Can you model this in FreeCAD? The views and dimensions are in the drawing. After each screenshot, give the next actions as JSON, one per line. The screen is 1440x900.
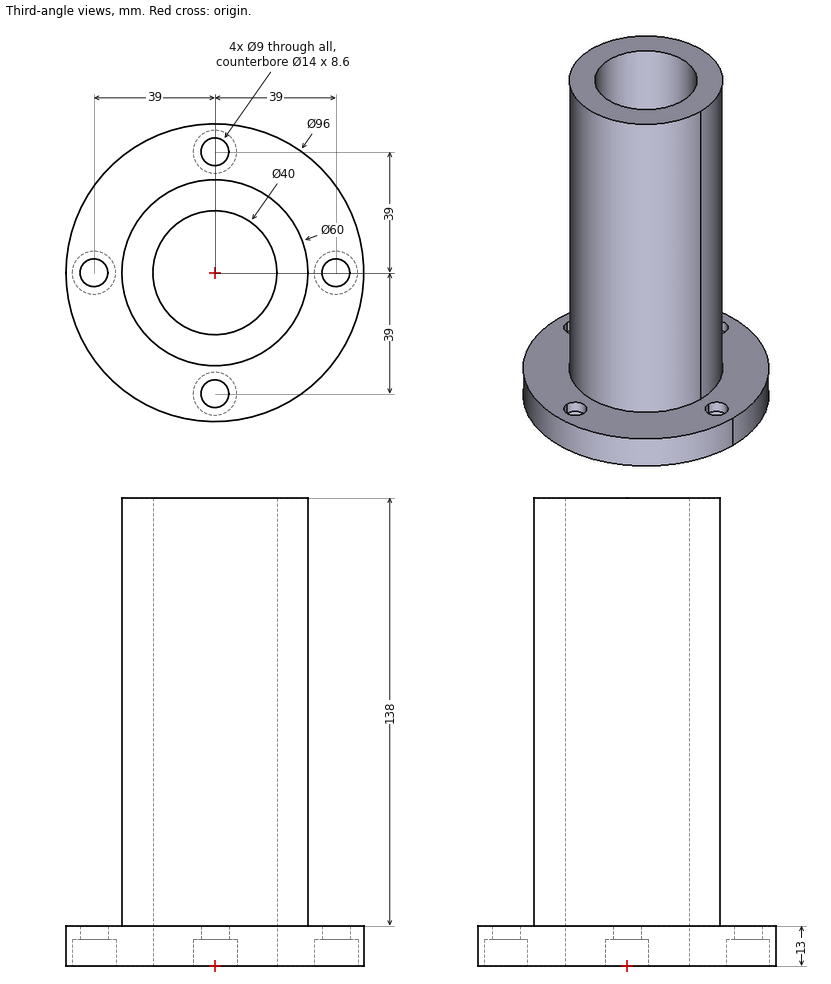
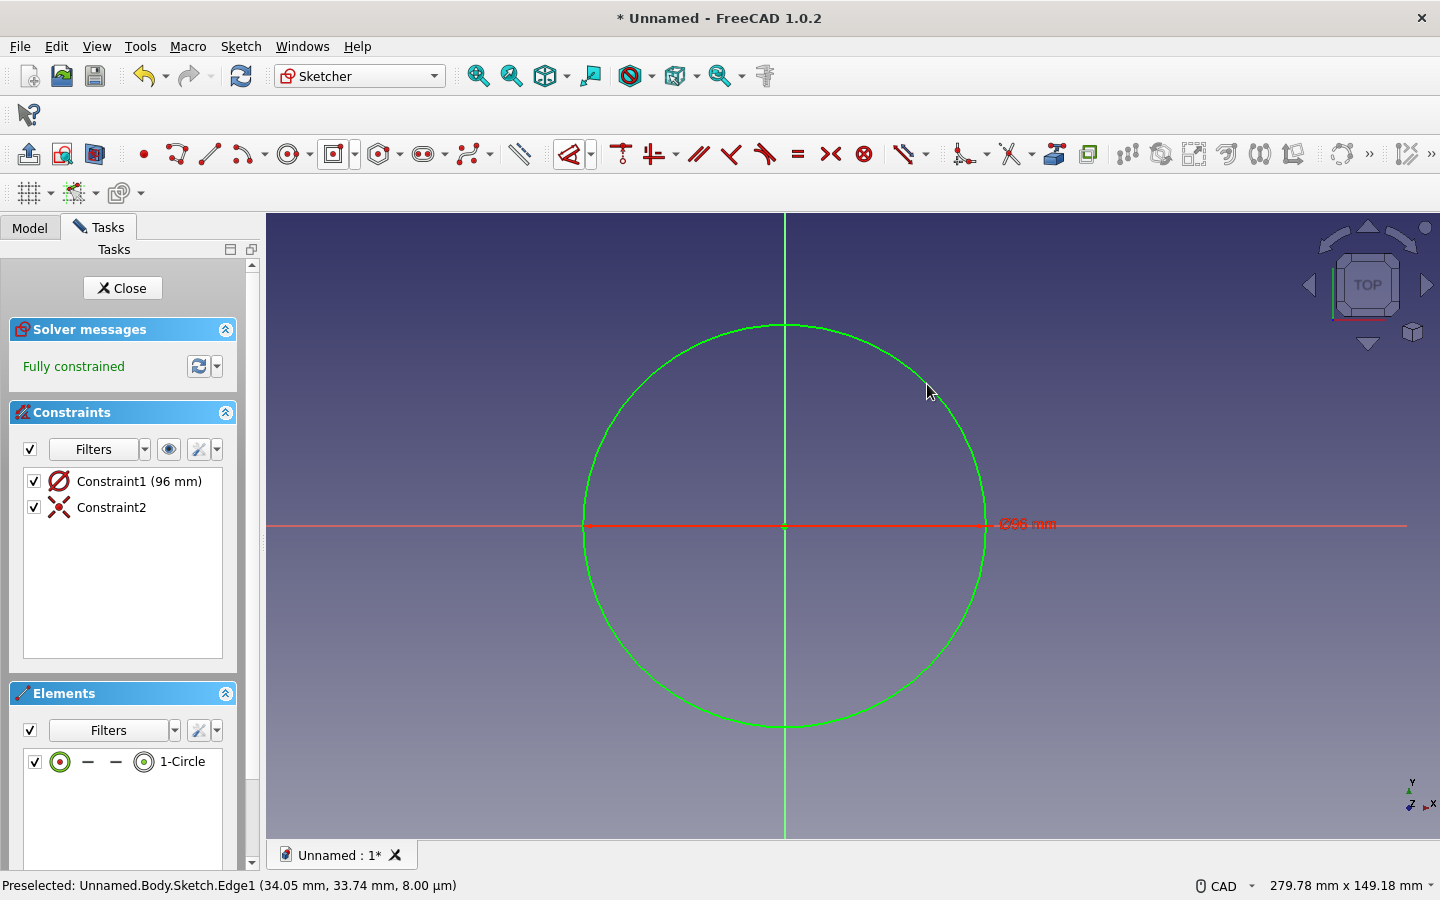
{"action": "left_click", "coordinate": [123, 288]}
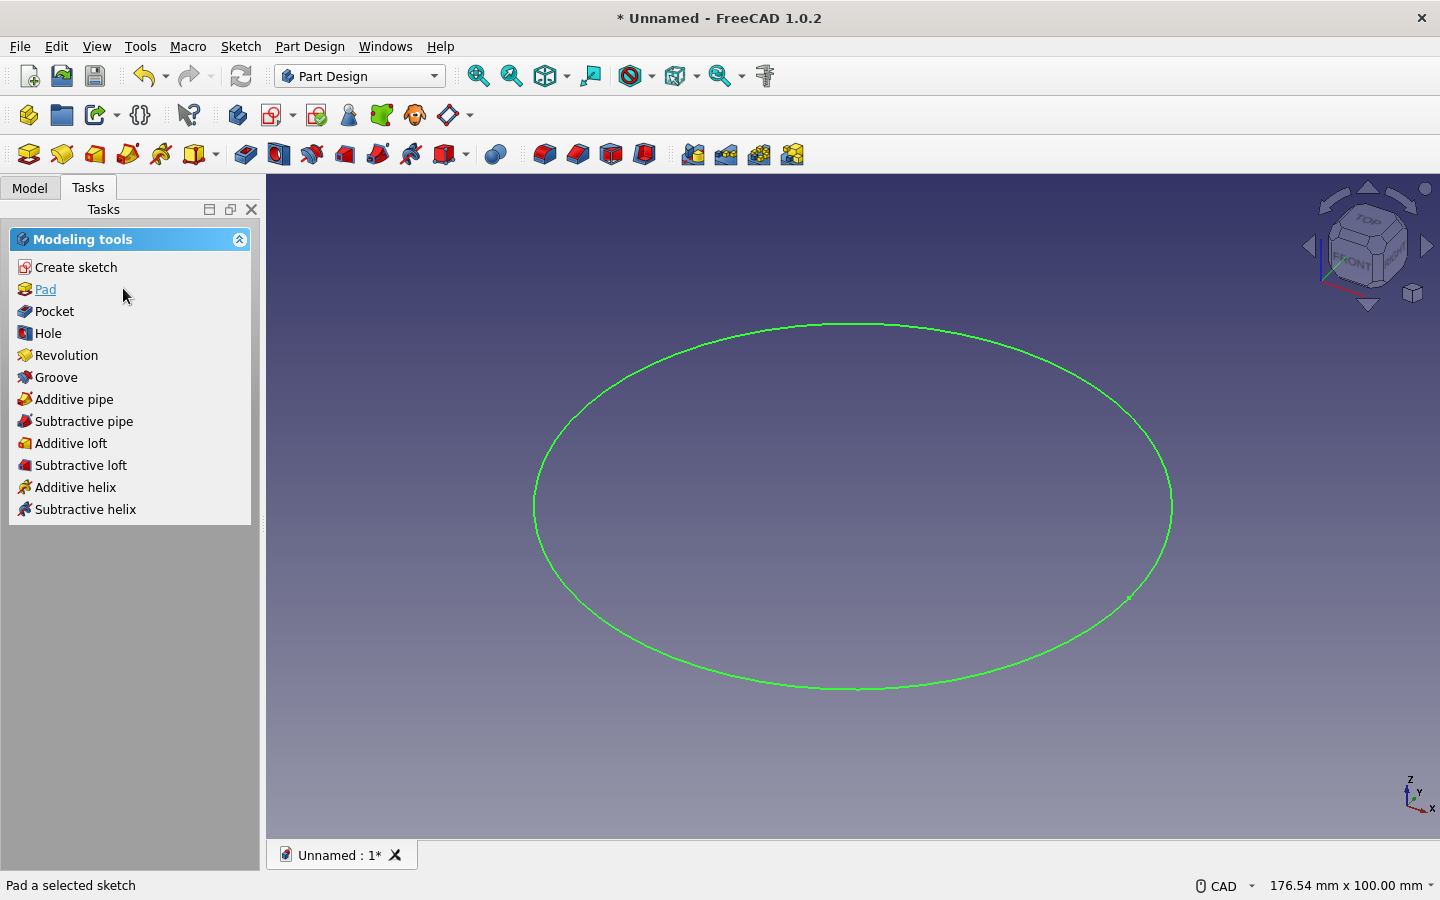
{"action": "left_click", "coordinate": [29, 154]}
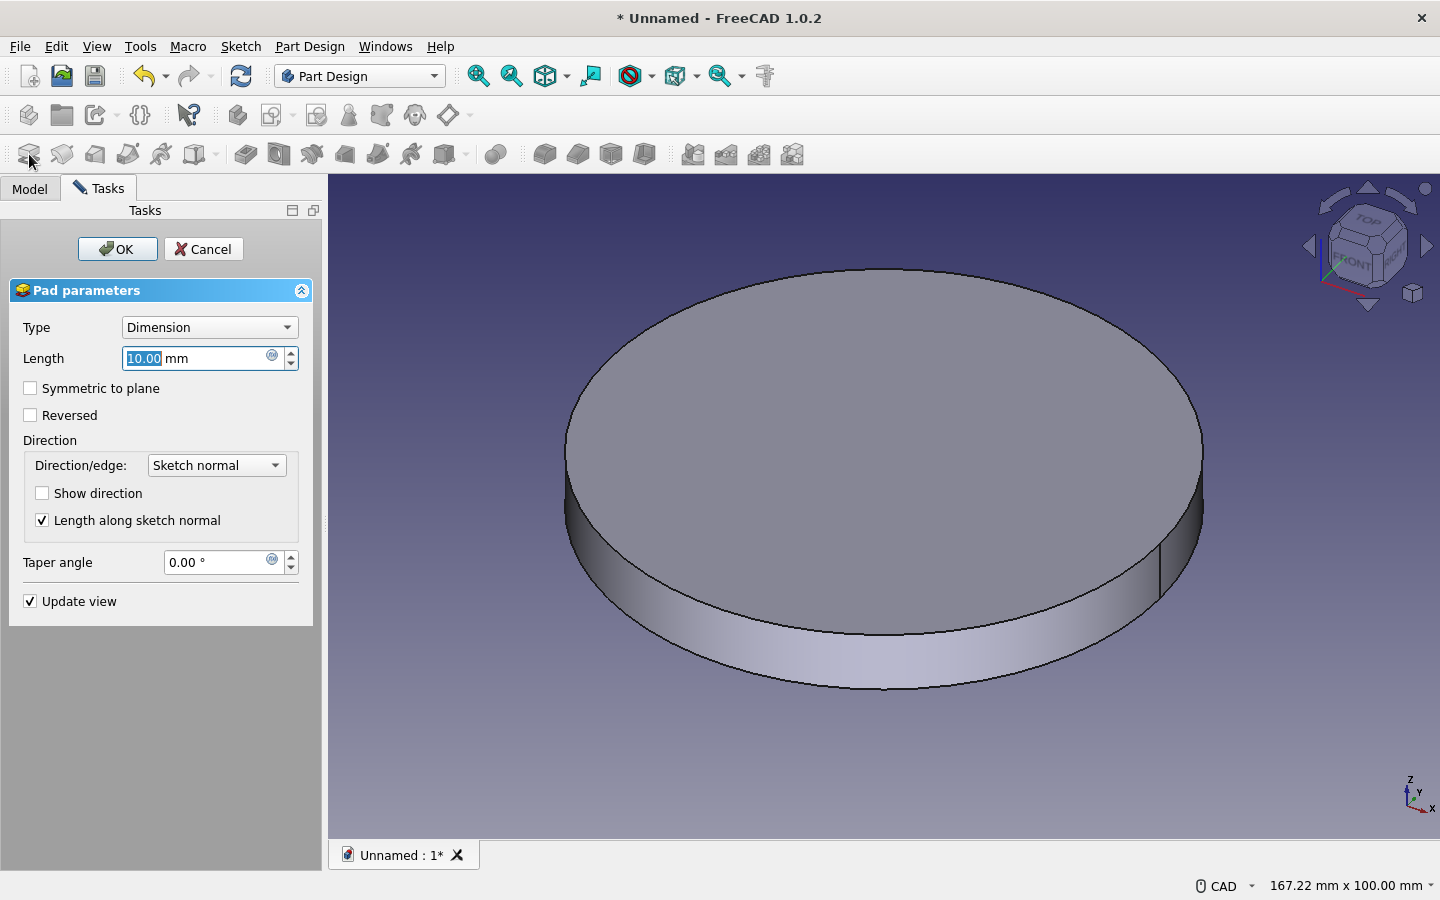
{"action": "type", "text": "13"}
{"action": "key", "text": "Tab"}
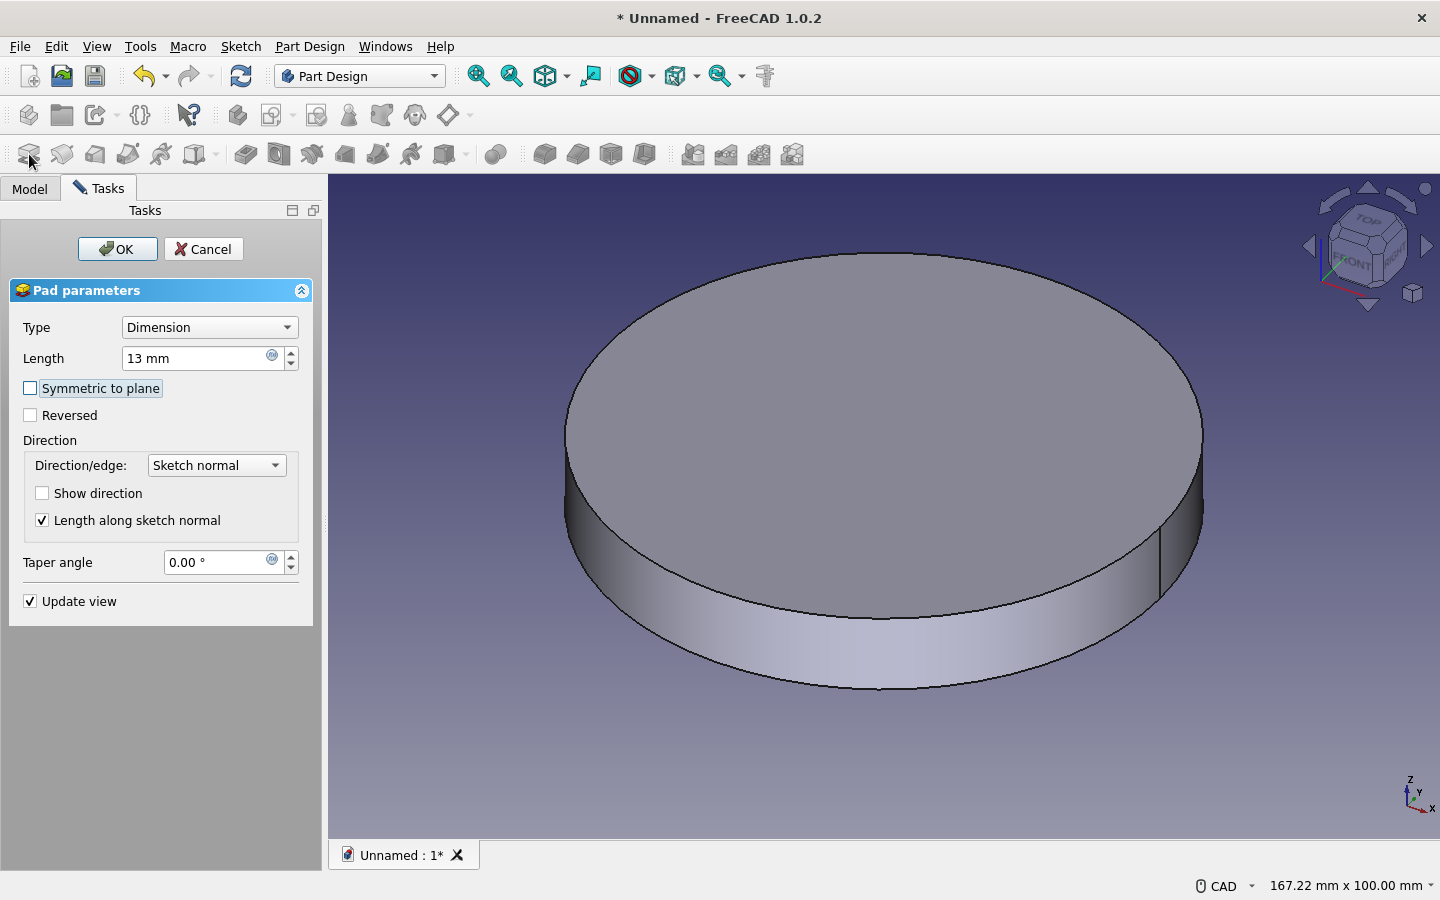
{"action": "left_click", "coordinate": [118, 249]}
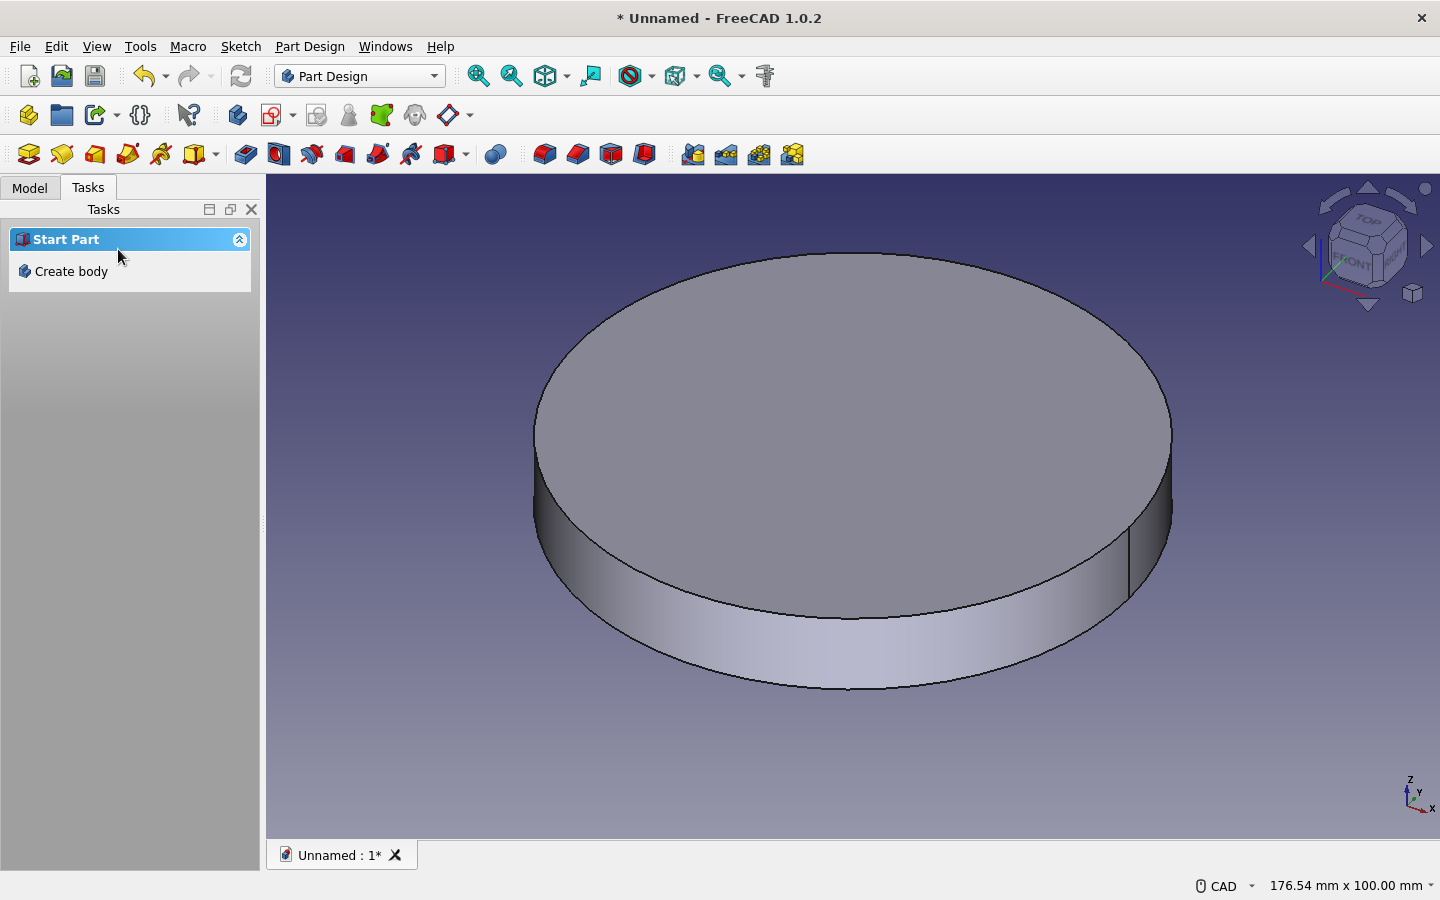
{"action": "left_click", "coordinate": [270, 116]}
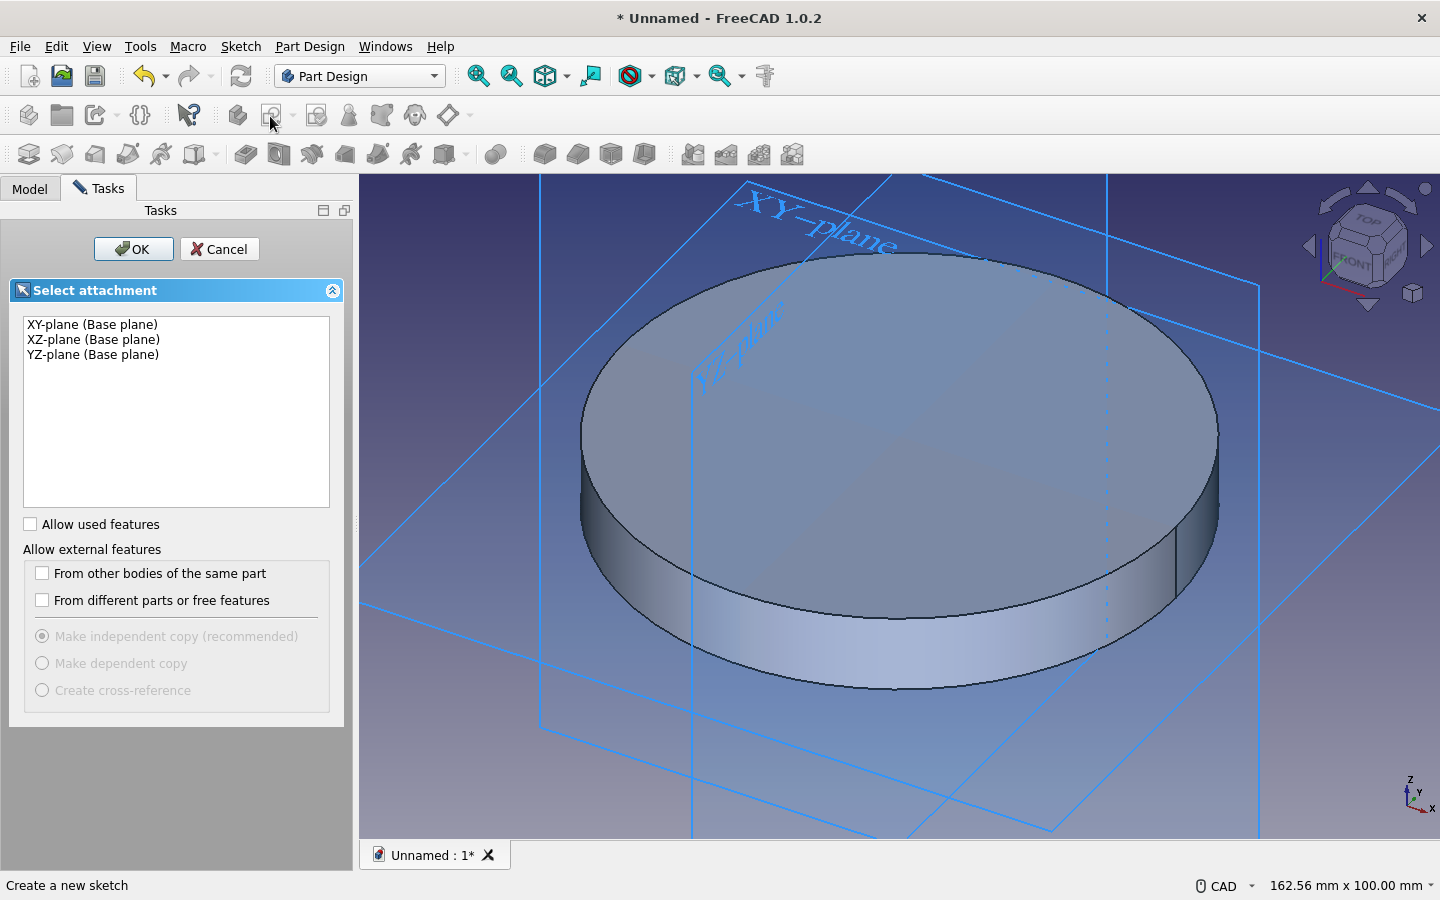
{"action": "left_click", "coordinate": [84, 324]}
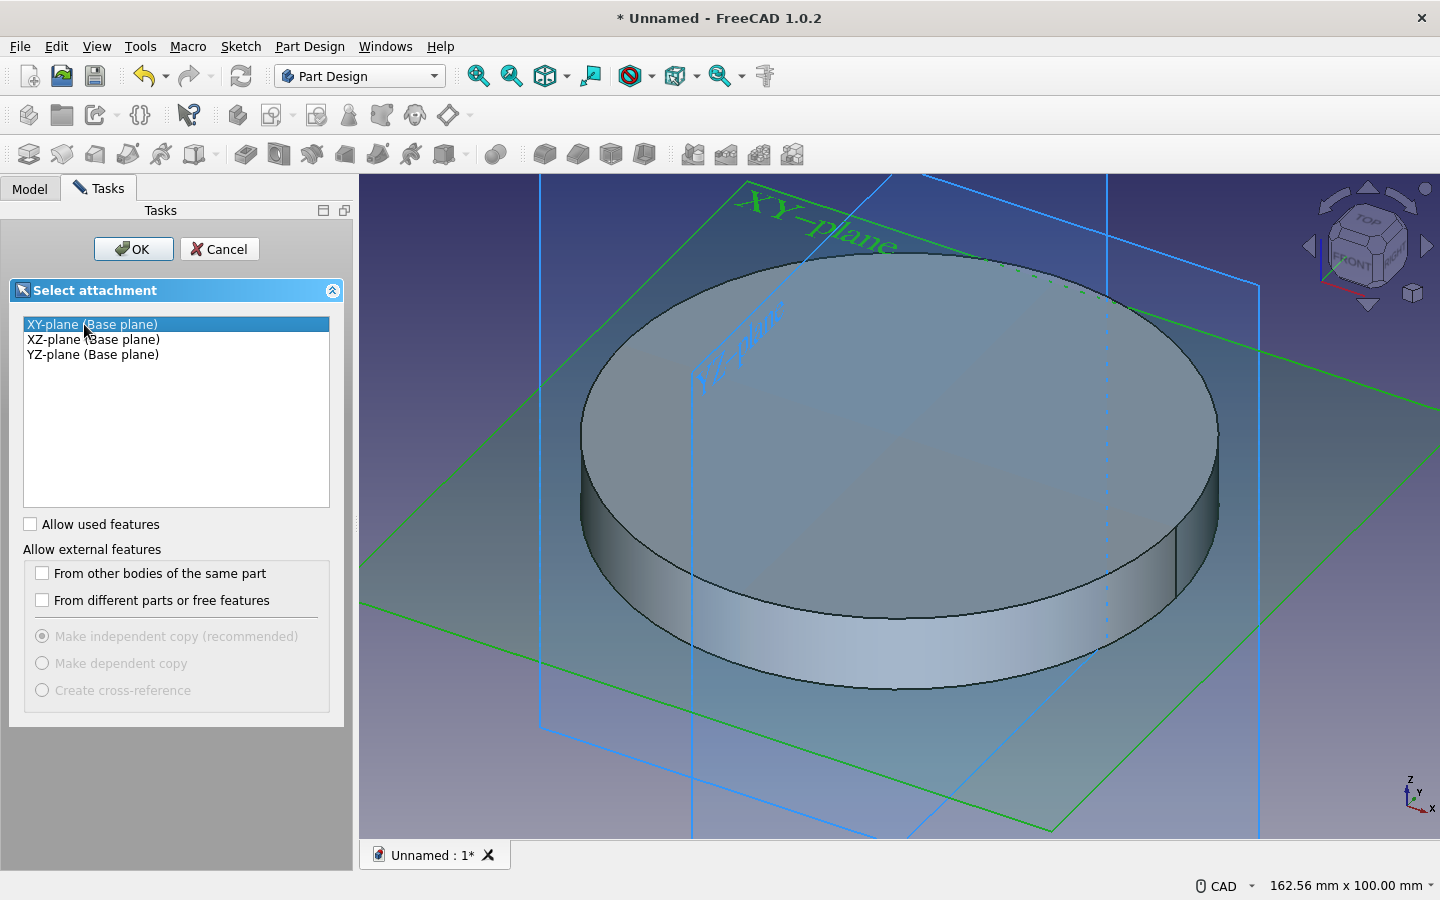
{"action": "left_click", "coordinate": [134, 249]}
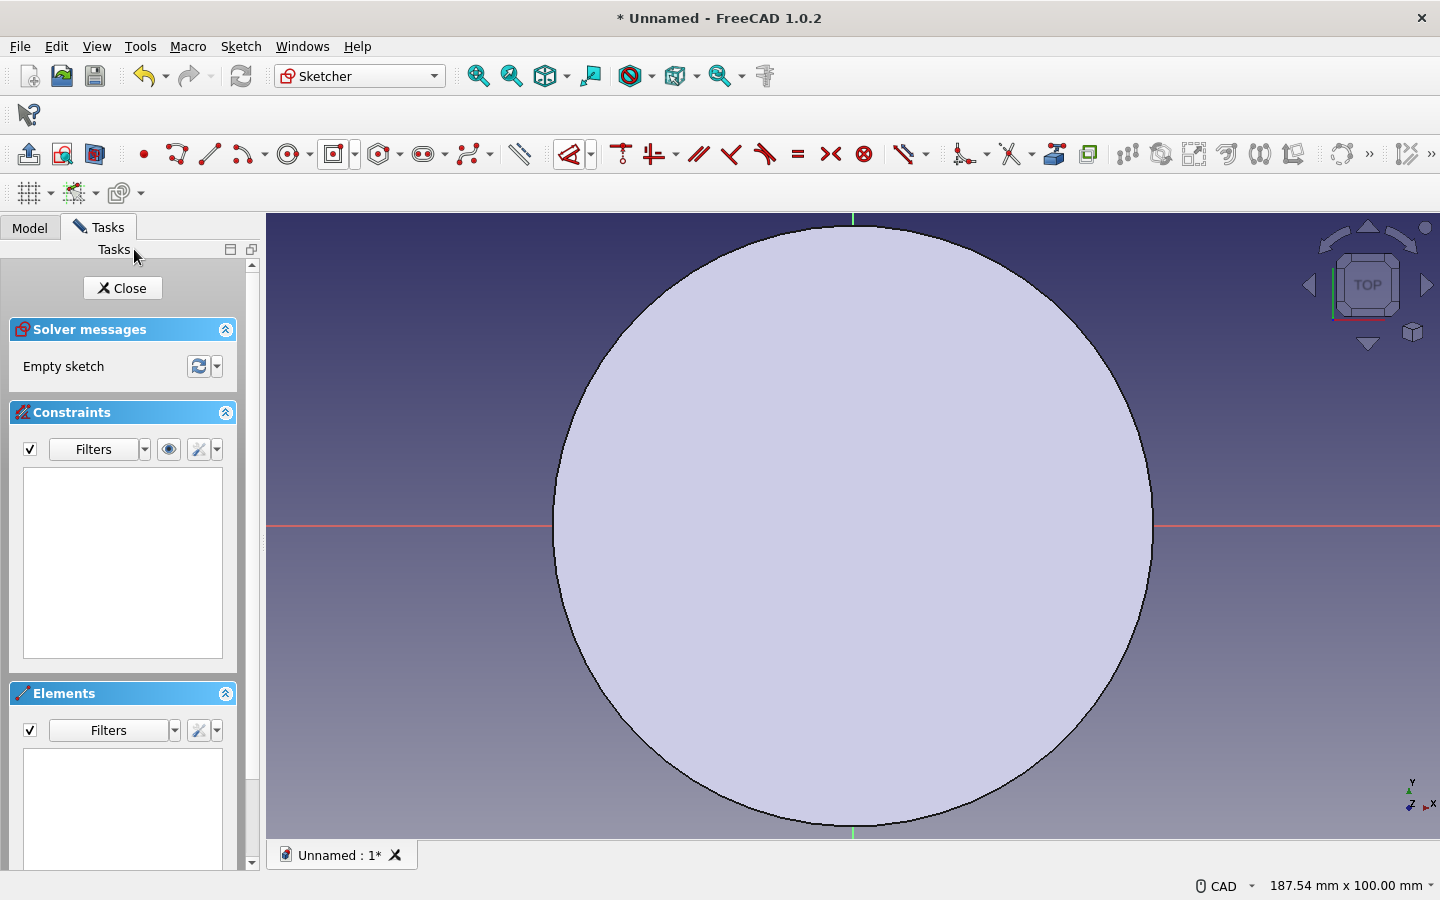
{"action": "key", "text": "q s"}